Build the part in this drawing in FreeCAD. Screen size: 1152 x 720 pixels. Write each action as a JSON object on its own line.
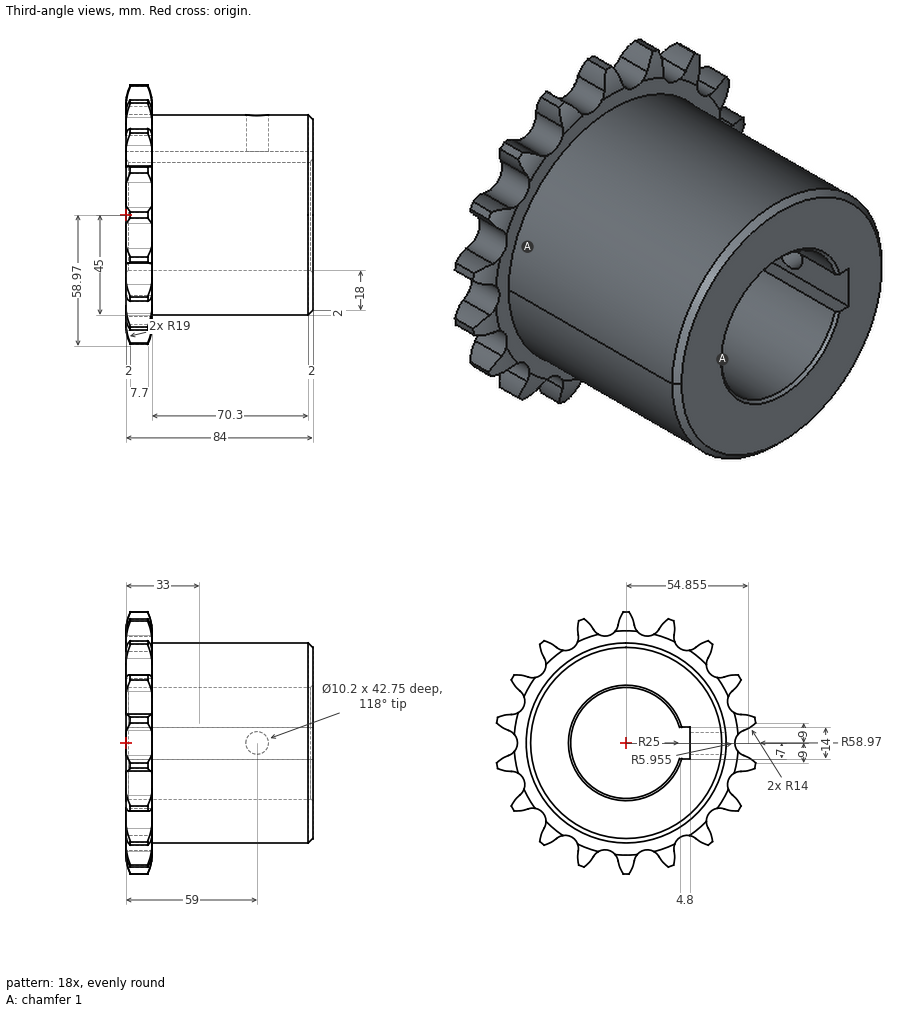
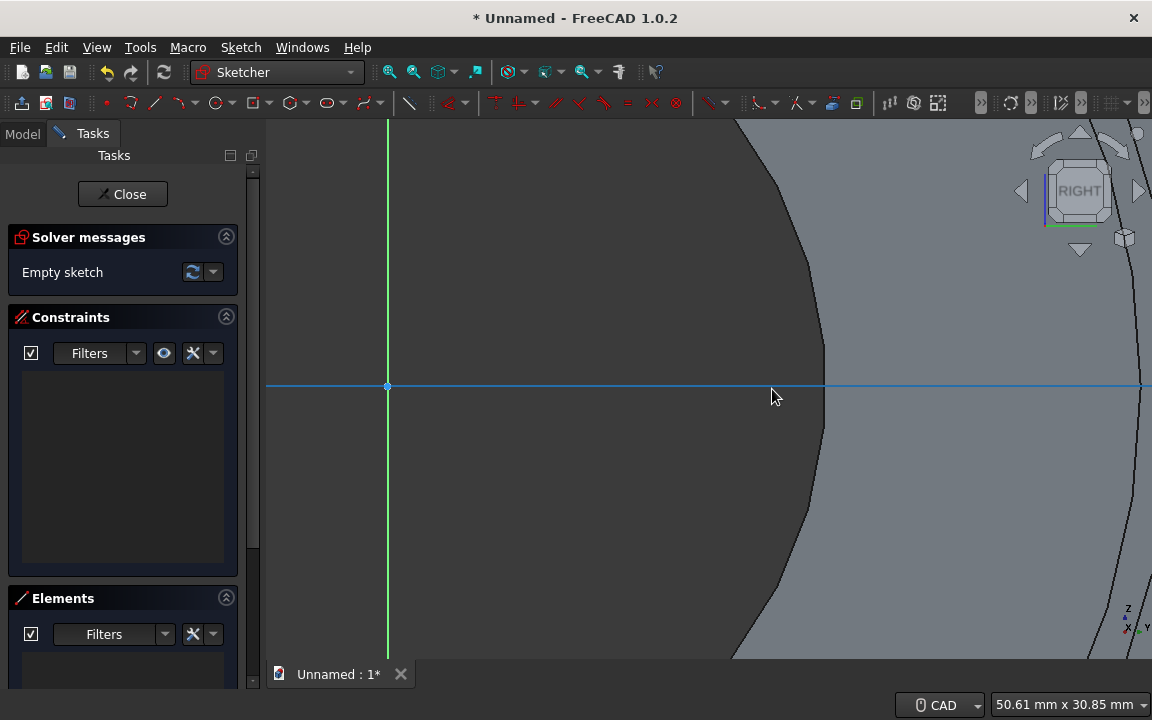
{"action": "key", "text": "g m"}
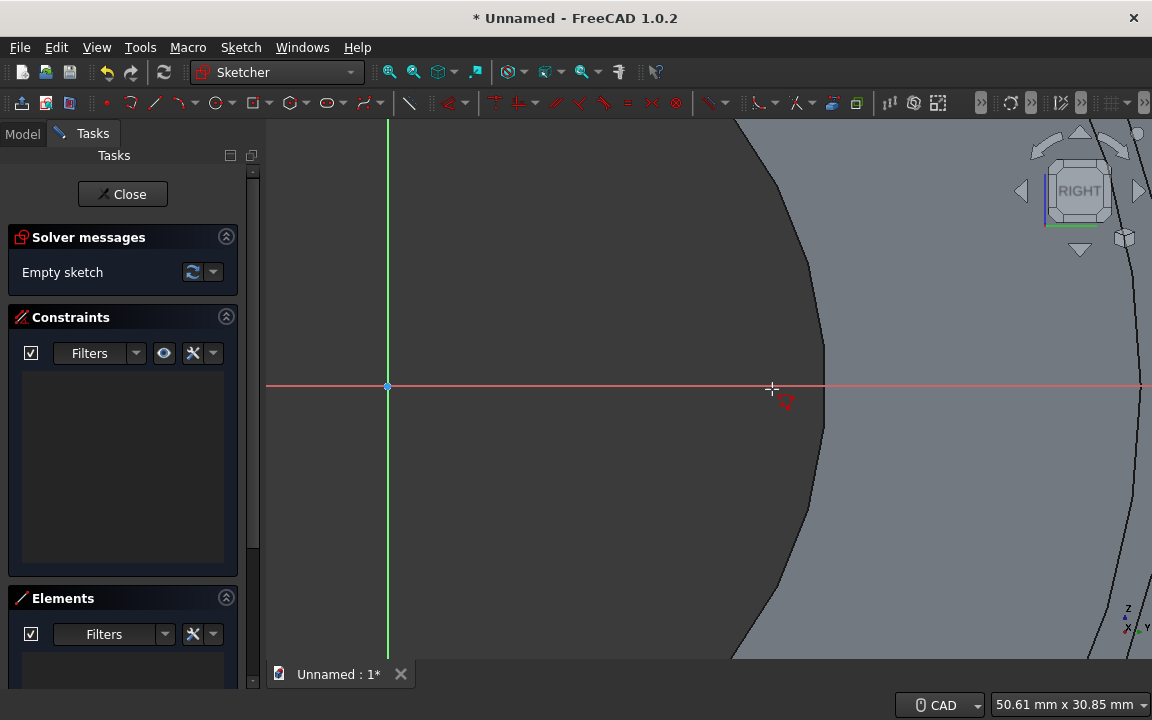
{"action": "left_click", "coordinate": [808, 509]}
{"action": "left_click", "coordinate": [892, 509]}
{"action": "left_click", "coordinate": [892, 264]}
{"action": "left_click", "coordinate": [808, 264]}
{"action": "right_click", "coordinate": [808, 264]}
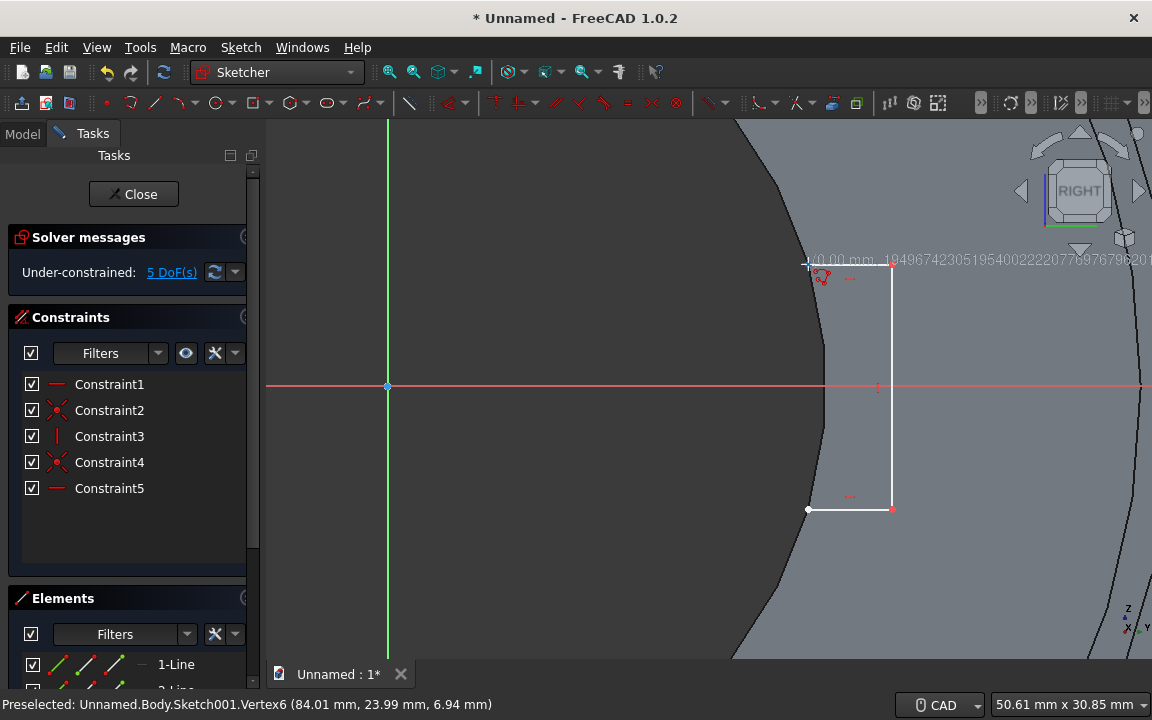
{"action": "key", "text": "g 3 a"}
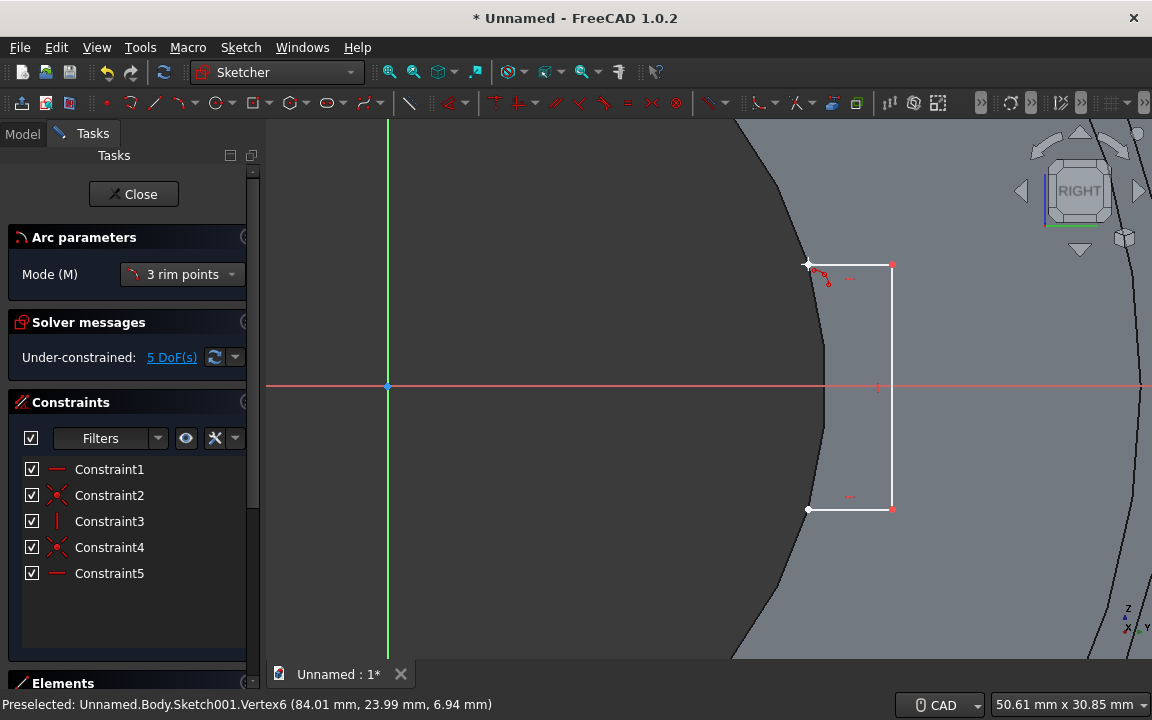
{"action": "left_click", "coordinate": [808, 265]}
{"action": "left_click", "coordinate": [808, 510]}
{"action": "left_click", "coordinate": [825, 411]}
{"action": "key", "text": "Escape"}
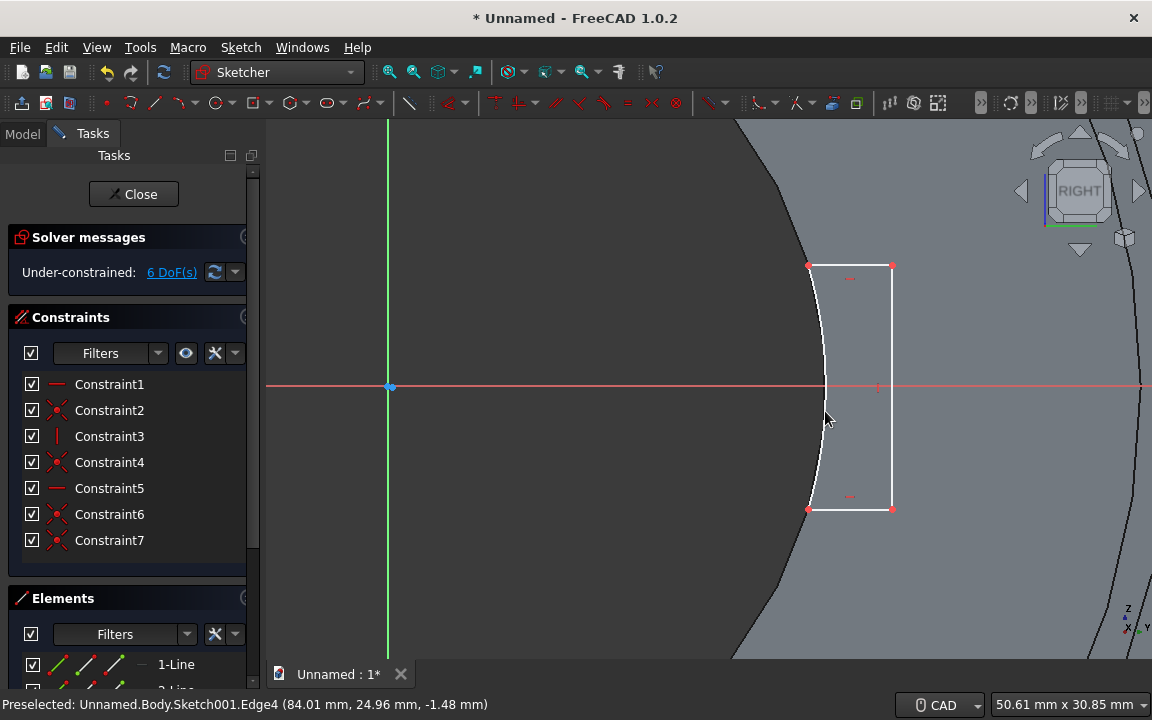
{"action": "left_click_drag", "start_coordinate": [378, 376], "coordinate": [403, 397]}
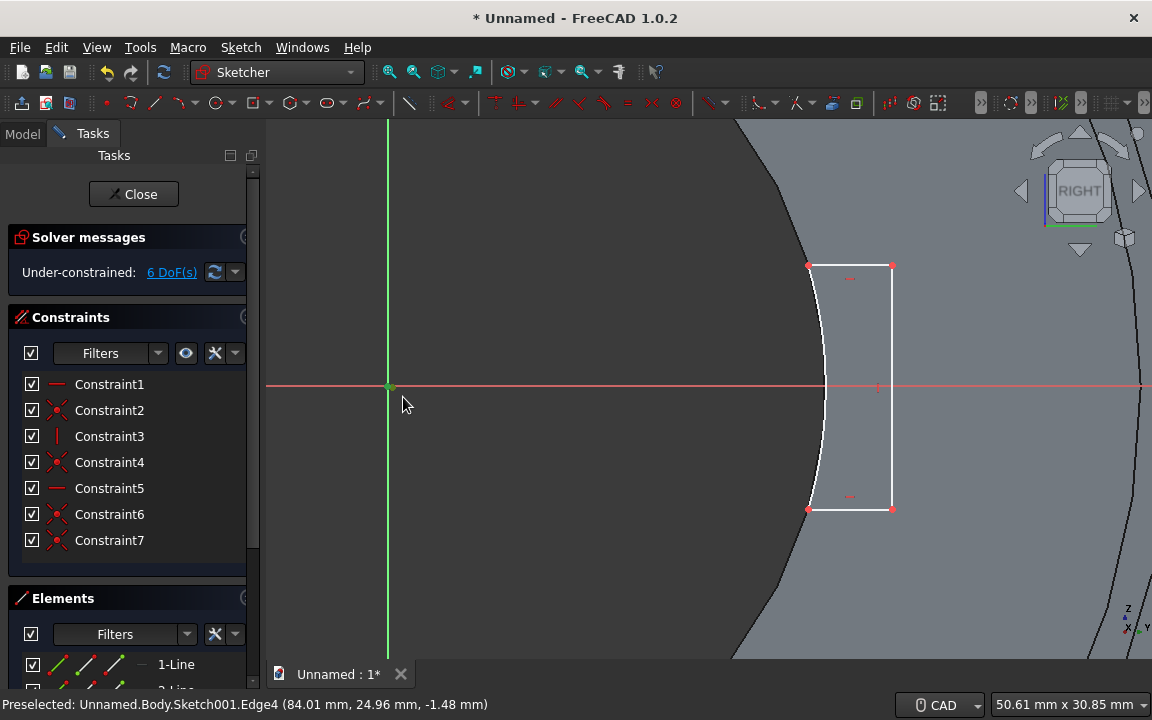
{"action": "key", "text": "c"}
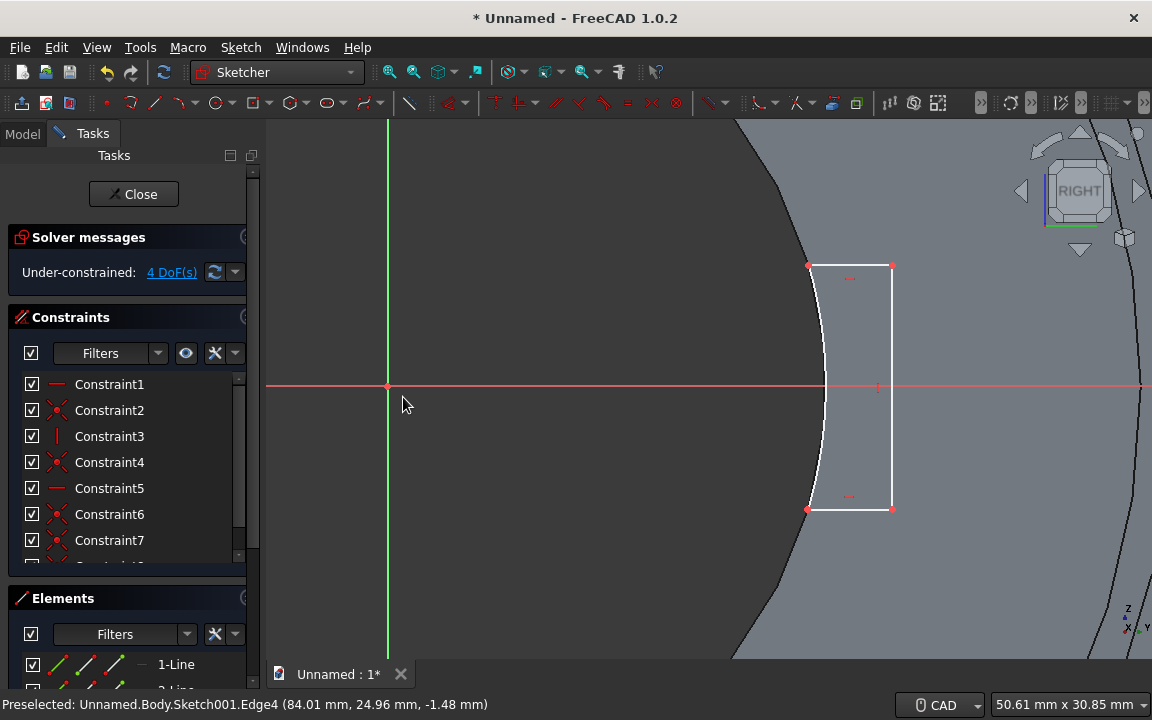
{"action": "key", "text": "d"}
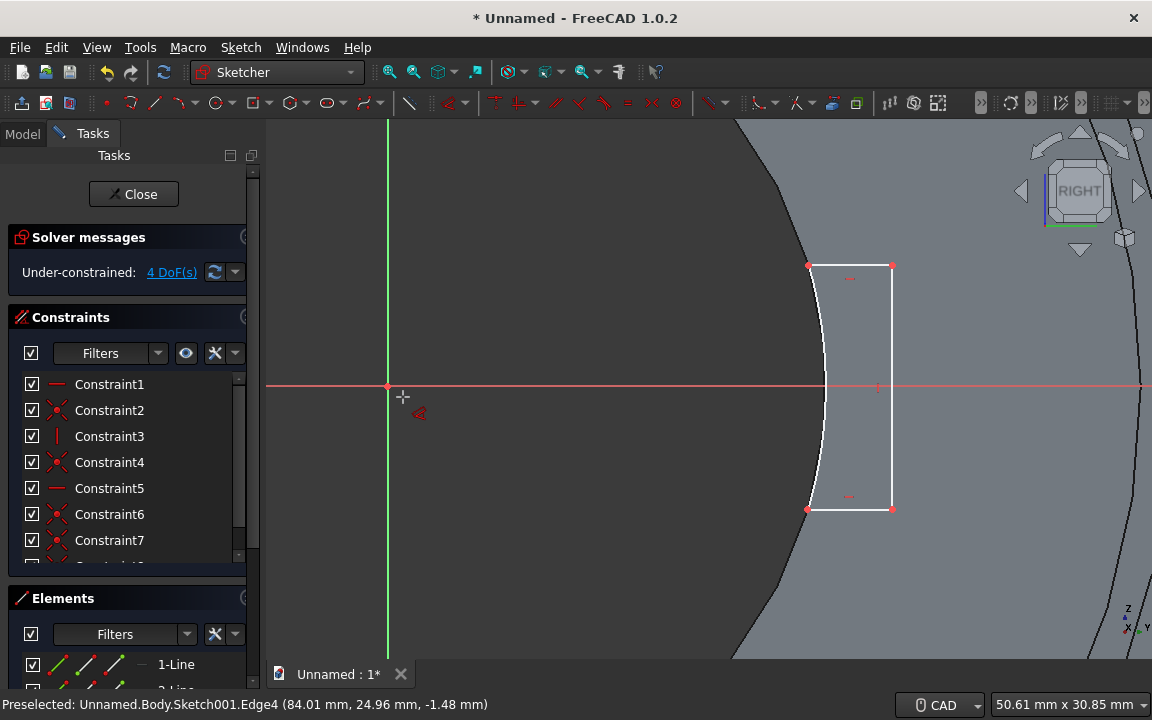
{"action": "left_click", "coordinate": [823, 437]}
{"action": "left_click", "coordinate": [855, 441]}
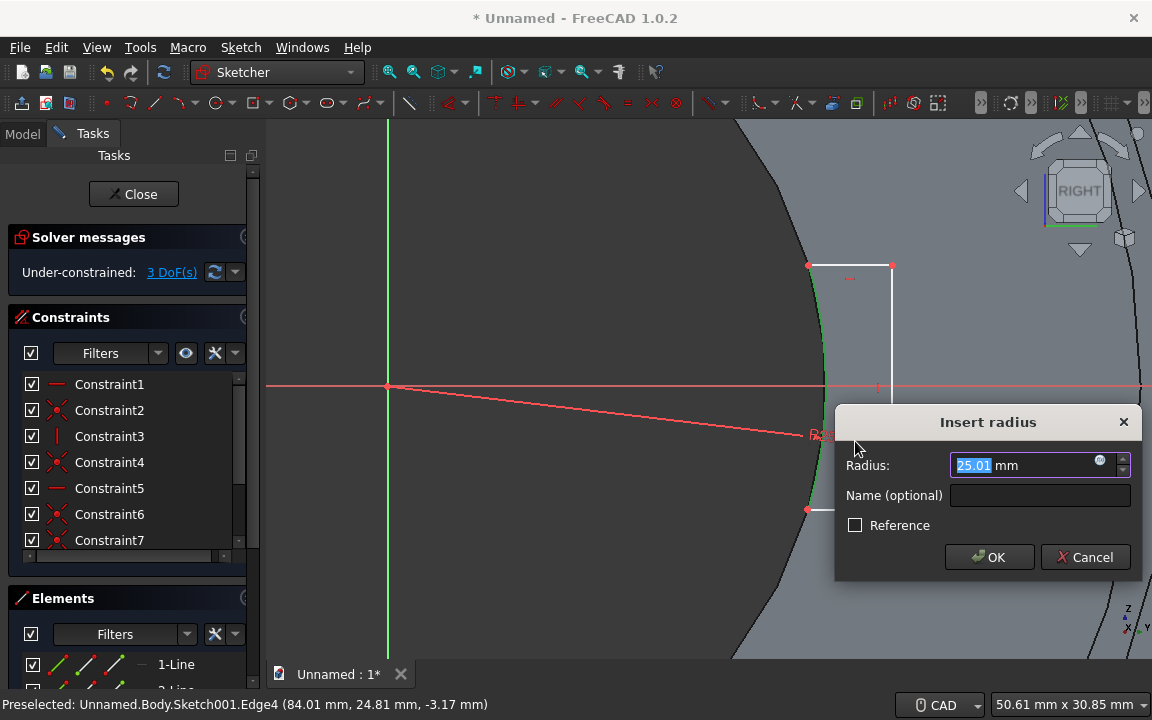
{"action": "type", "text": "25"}
{"action": "key", "text": "Return"}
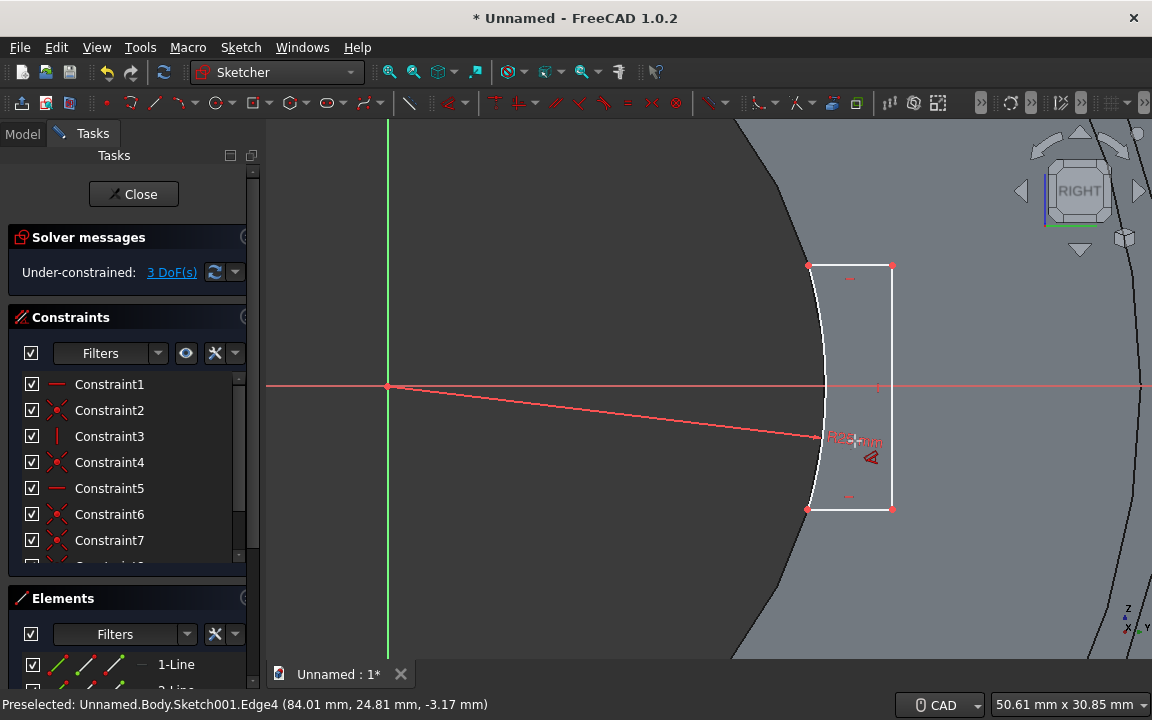
{"action": "left_click", "coordinate": [892, 437]}
{"action": "left_click", "coordinate": [926, 331]}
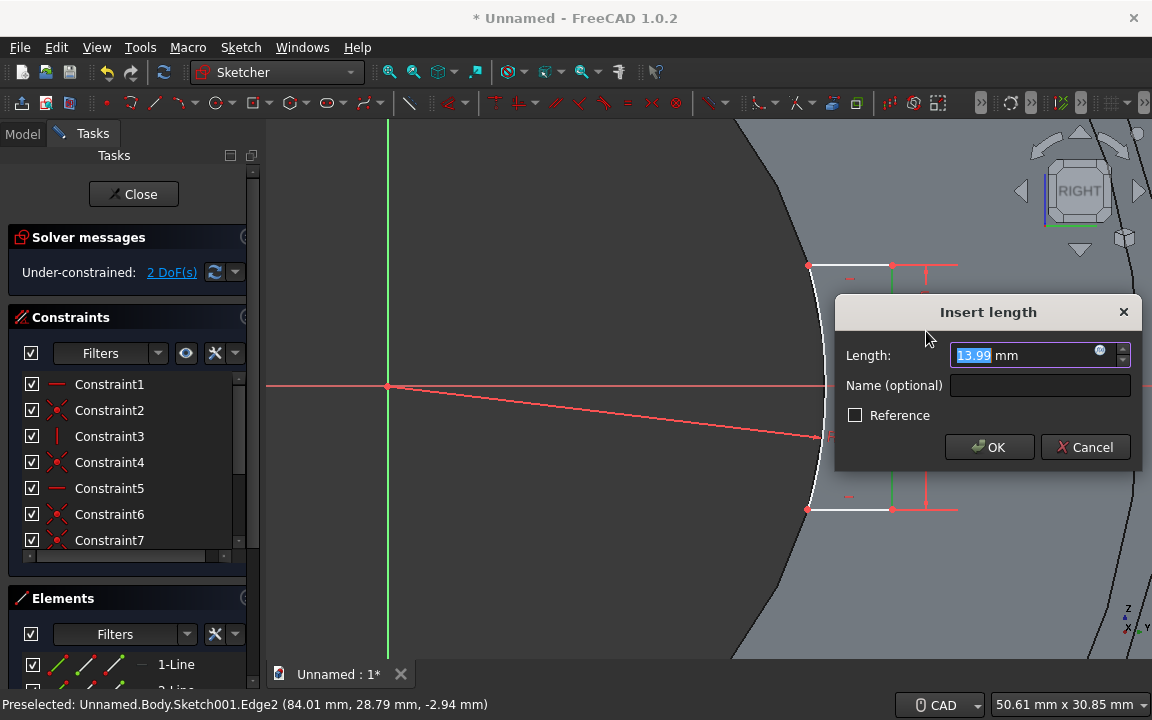
{"action": "type", "text": "14"}
{"action": "key", "text": "Return"}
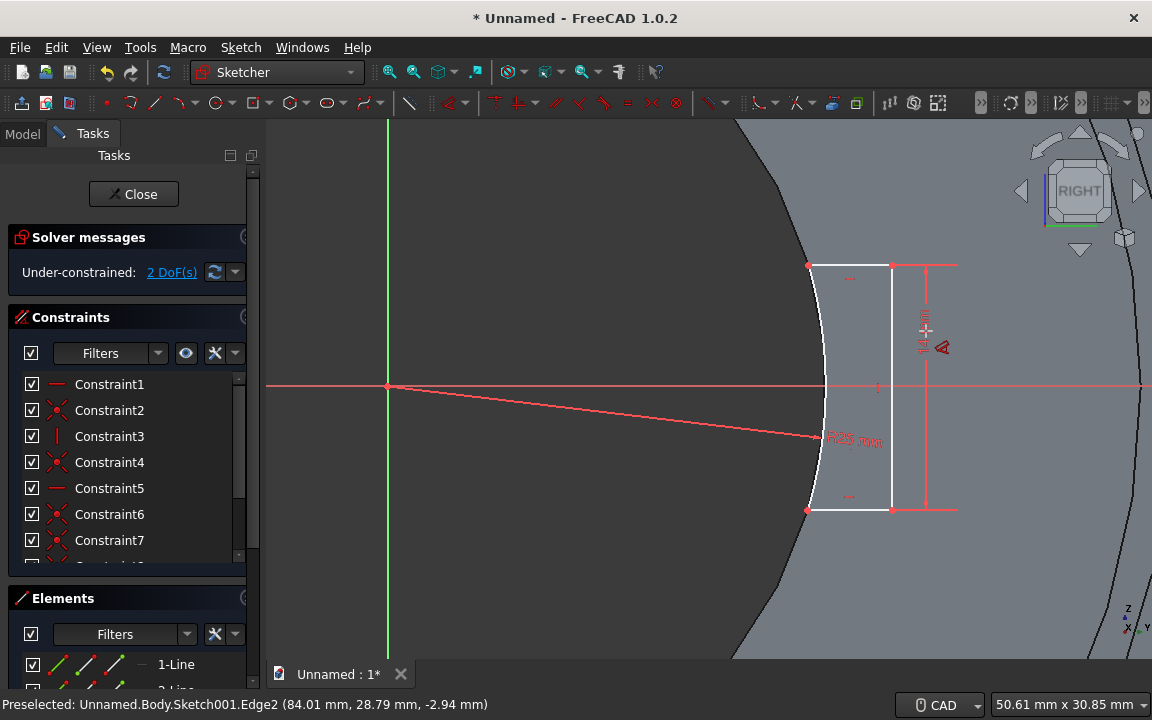
{"action": "left_click", "coordinate": [808, 510]}
{"action": "left_click", "coordinate": [354, 448]}